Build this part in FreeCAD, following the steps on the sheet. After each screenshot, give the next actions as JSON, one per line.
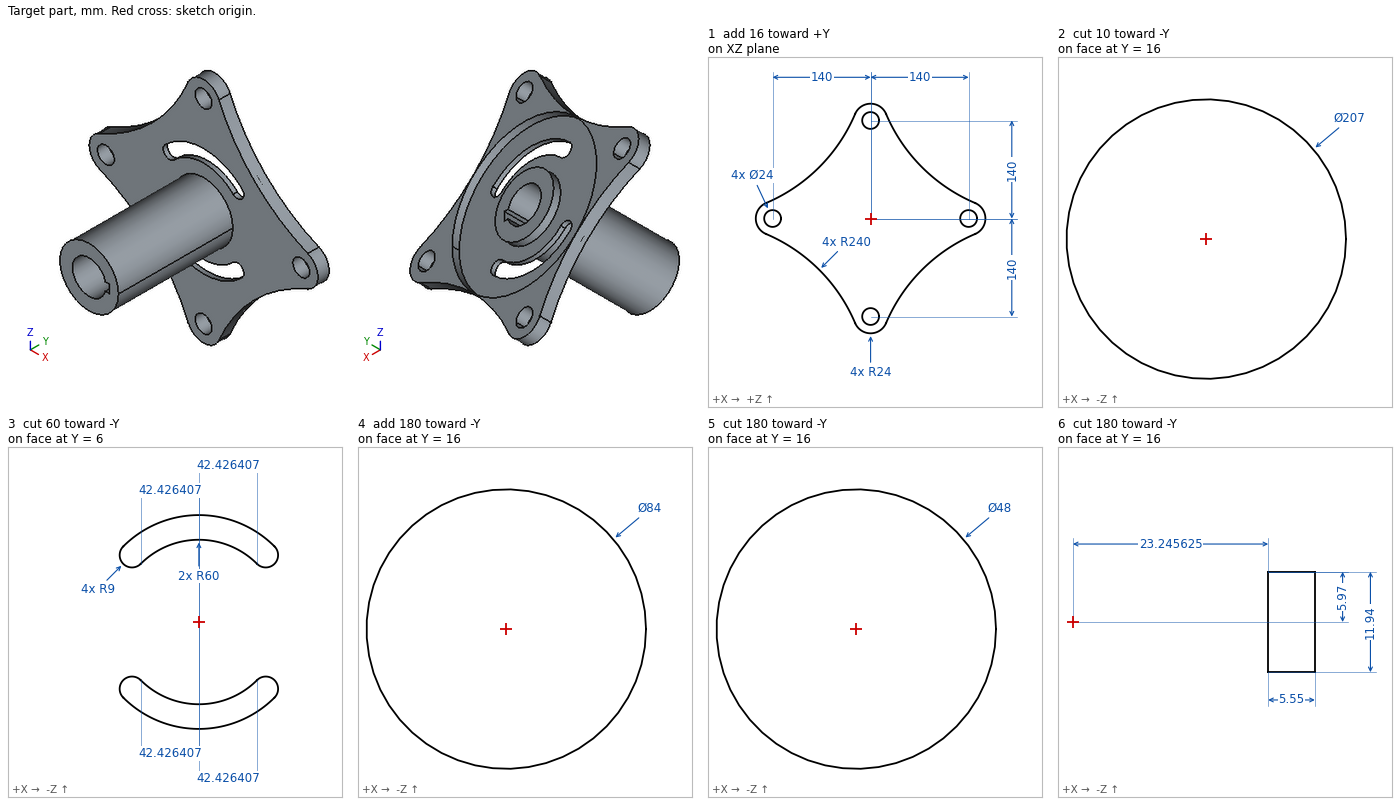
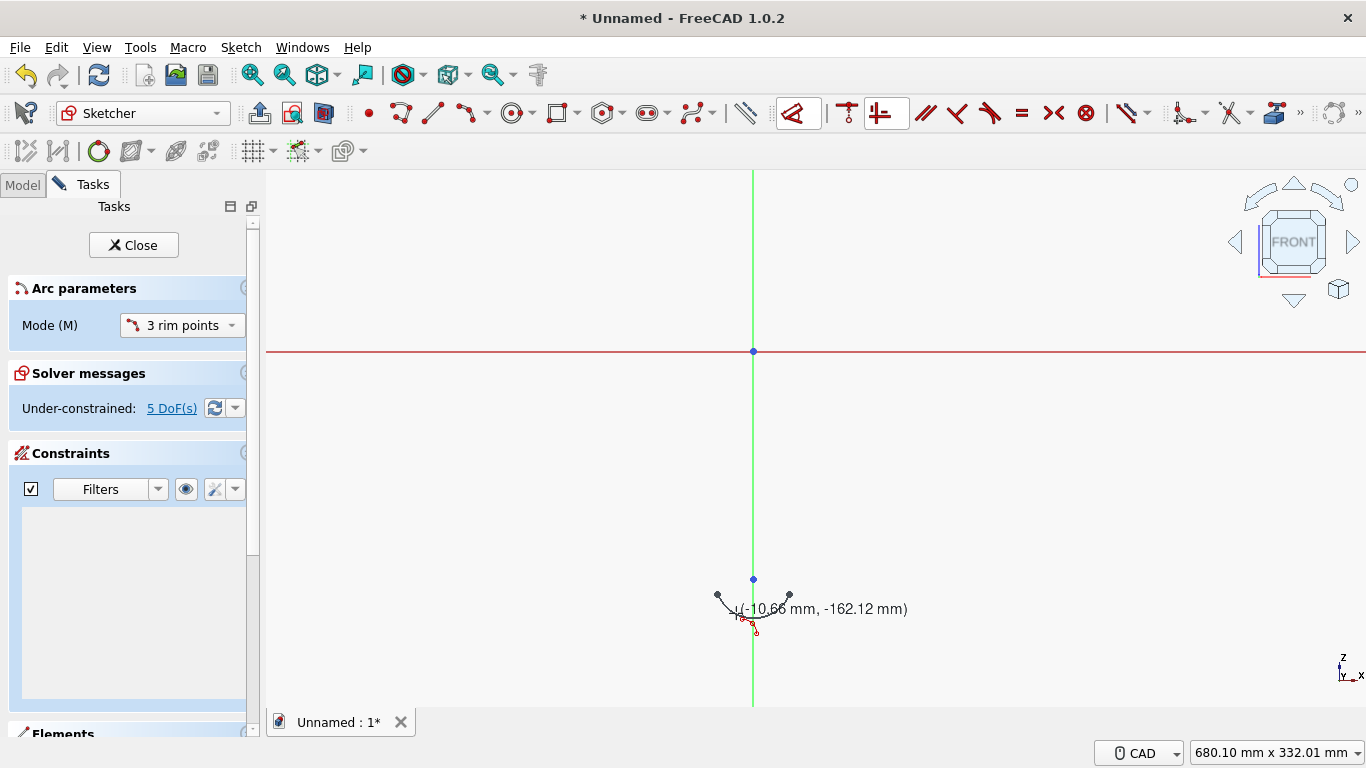
{"action": "left_click", "coordinate": [718, 594]}
{"action": "left_click", "coordinate": [512, 388]}
{"action": "left_click", "coordinate": [635, 470]}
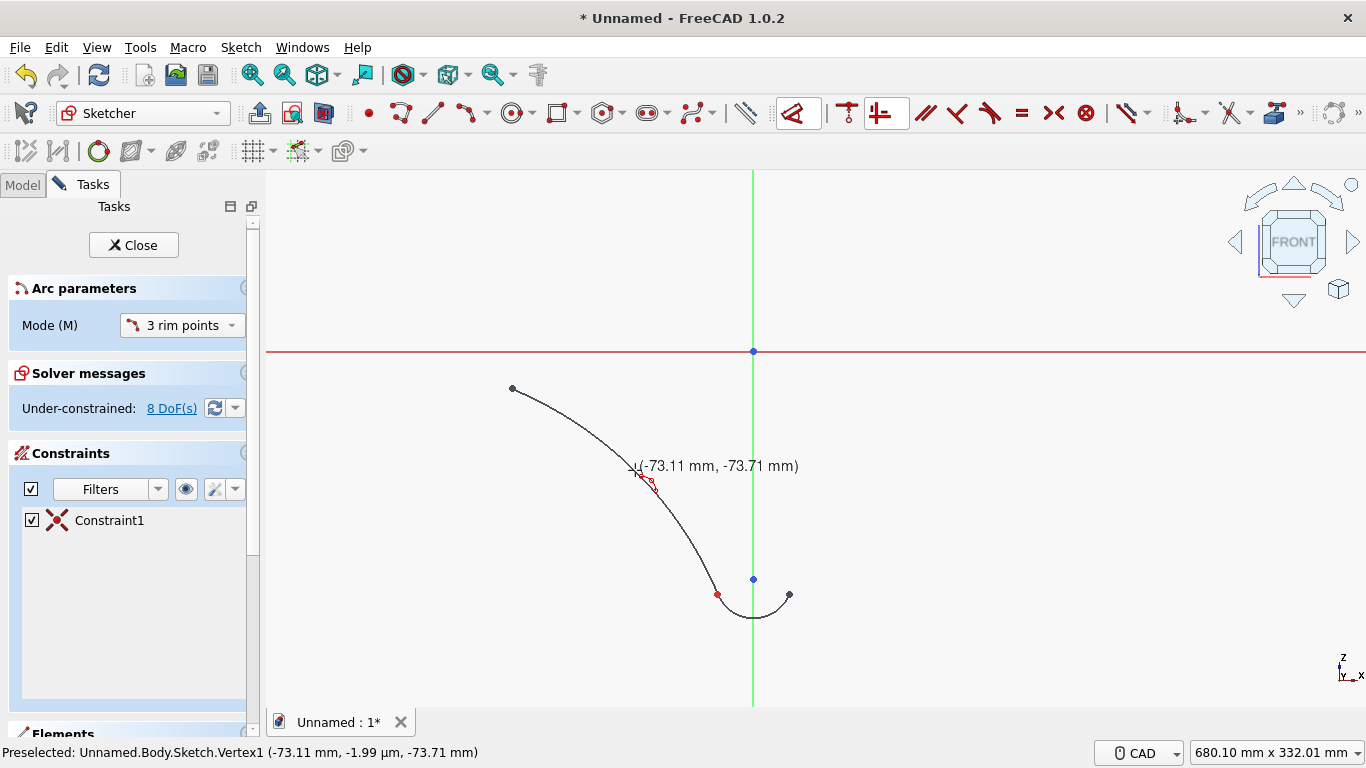
{"action": "left_click", "coordinate": [512, 389]}
{"action": "left_click", "coordinate": [512, 316]}
{"action": "left_click", "coordinate": [492, 334]}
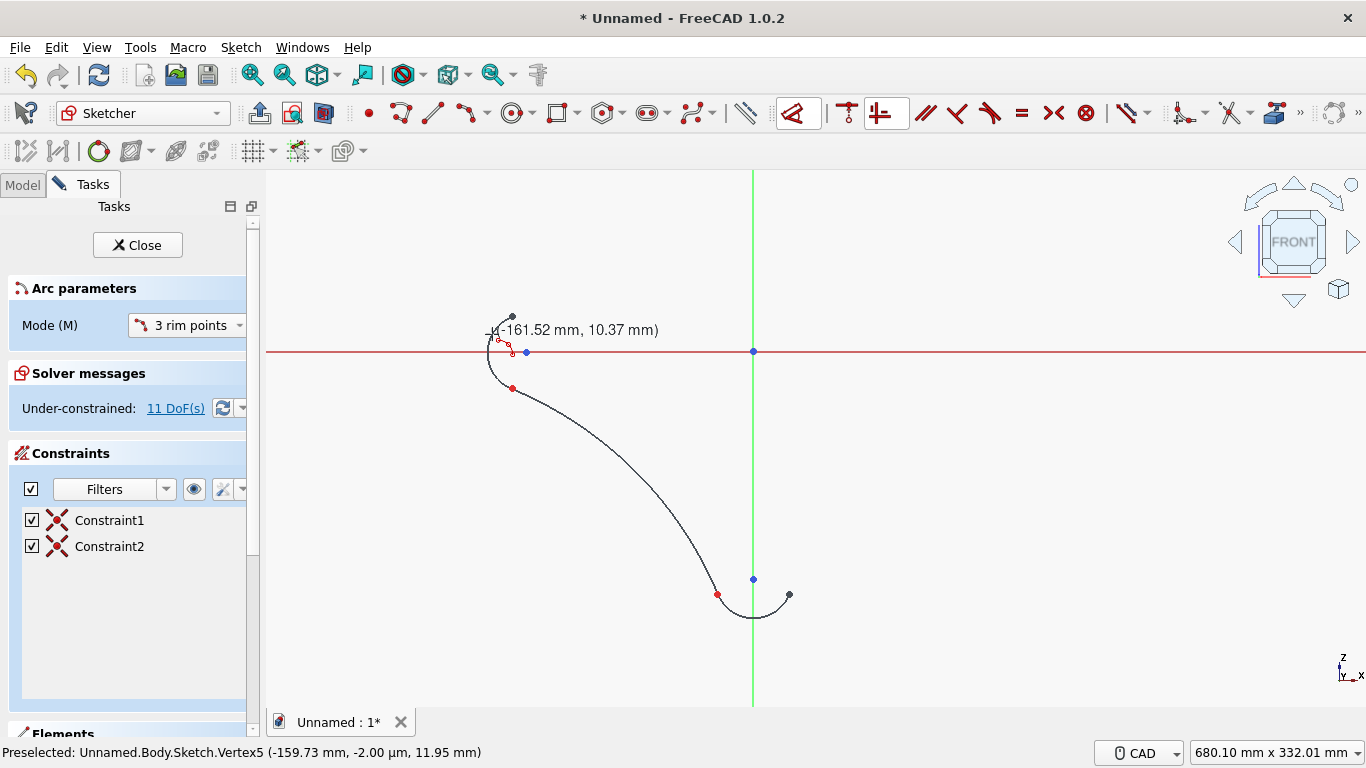
{"action": "left_click", "coordinate": [512, 317]}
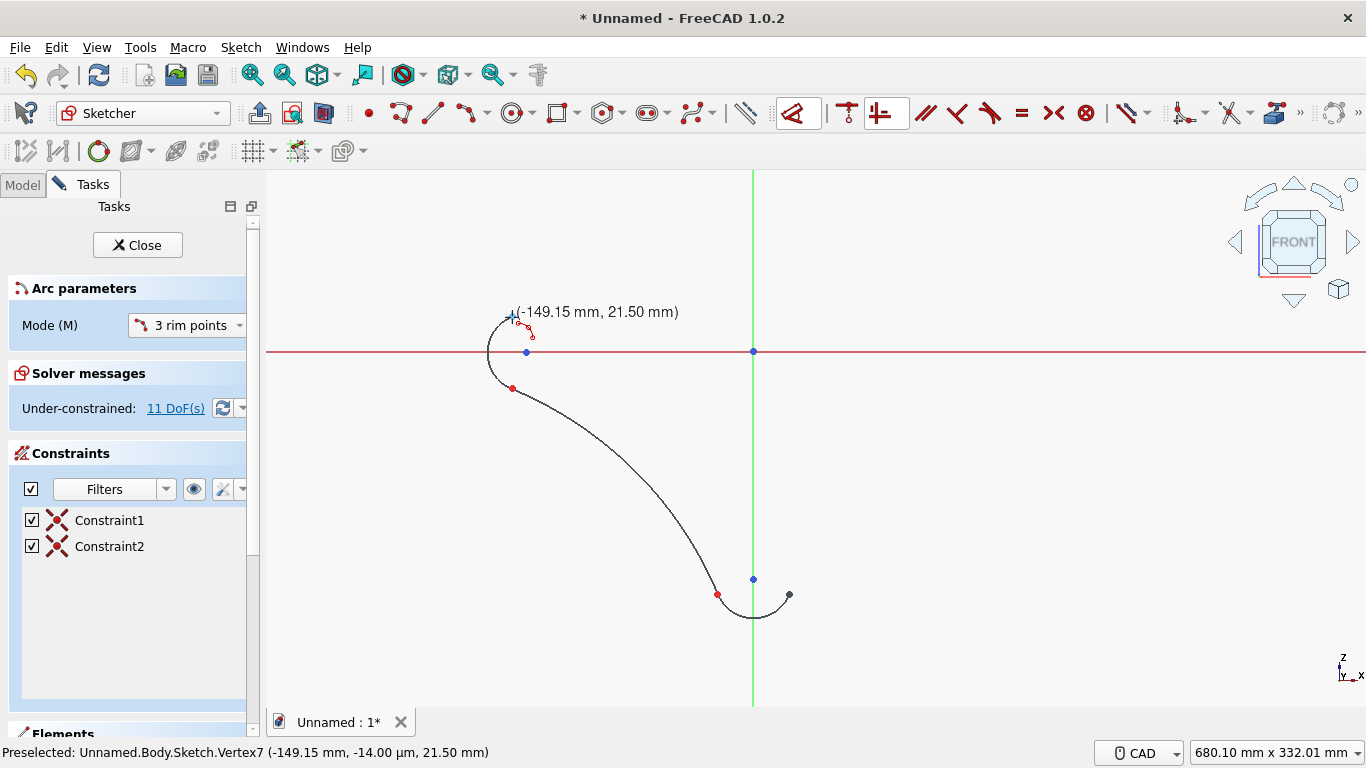
{"action": "scroll", "coordinate": [736, 615], "scroll_direction": "down", "scroll_amount": 2}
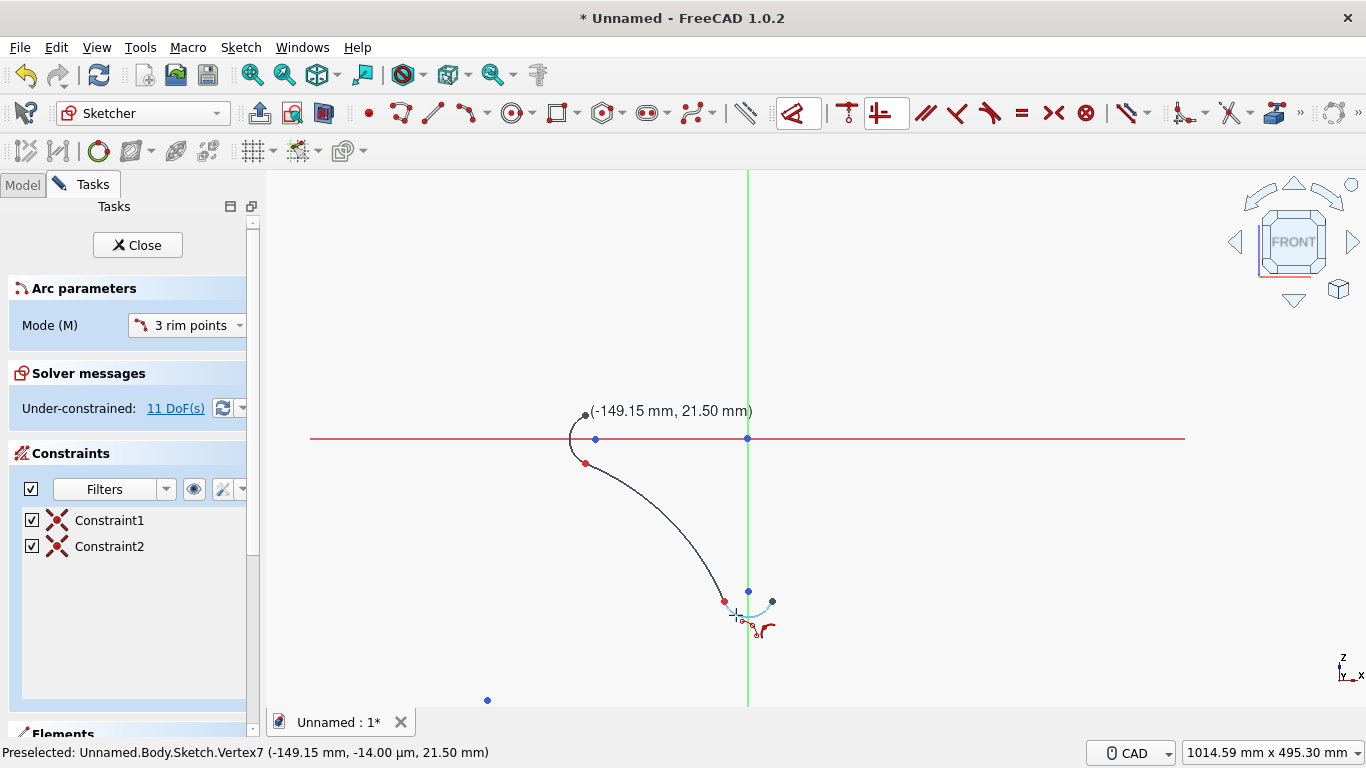
{"action": "left_click", "coordinate": [724, 277]}
{"action": "left_click", "coordinate": [668, 359]}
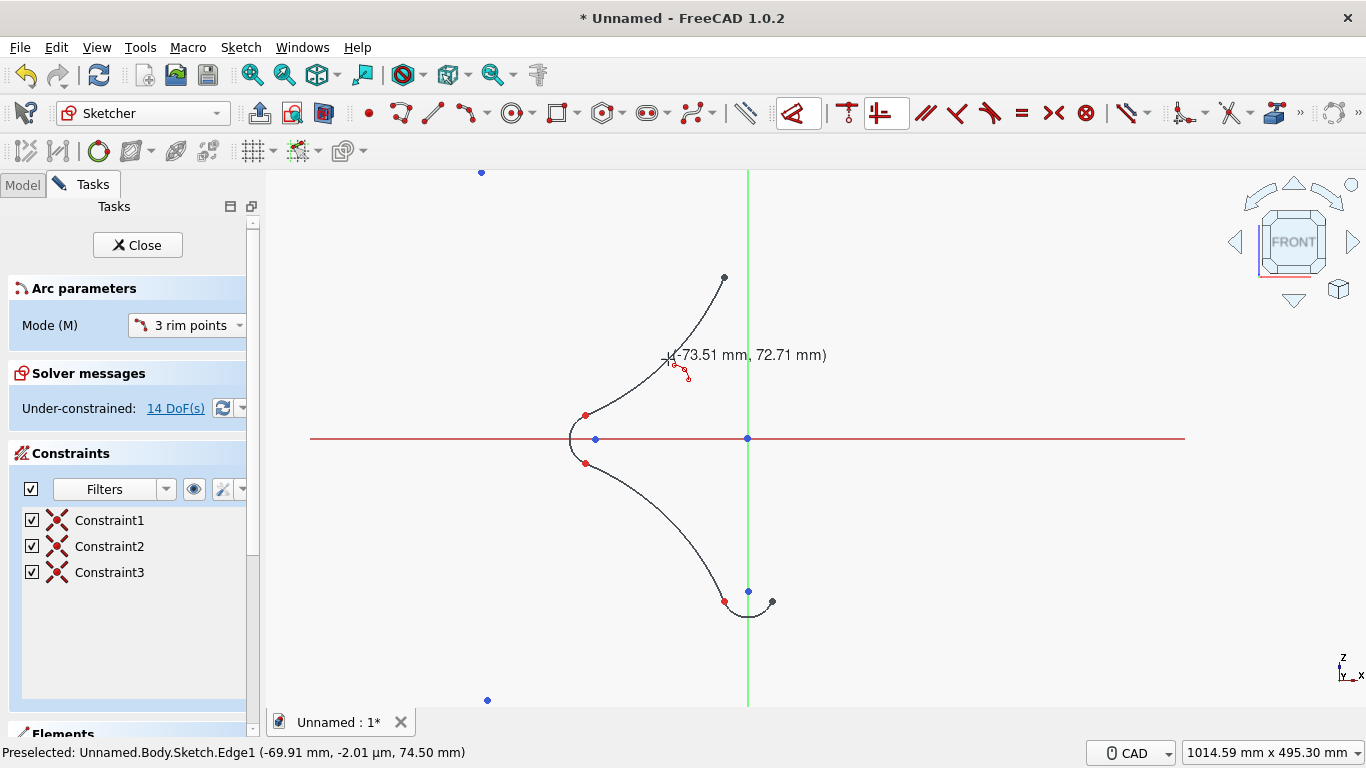
{"action": "left_click", "coordinate": [724, 278]}
{"action": "left_click", "coordinate": [772, 277]}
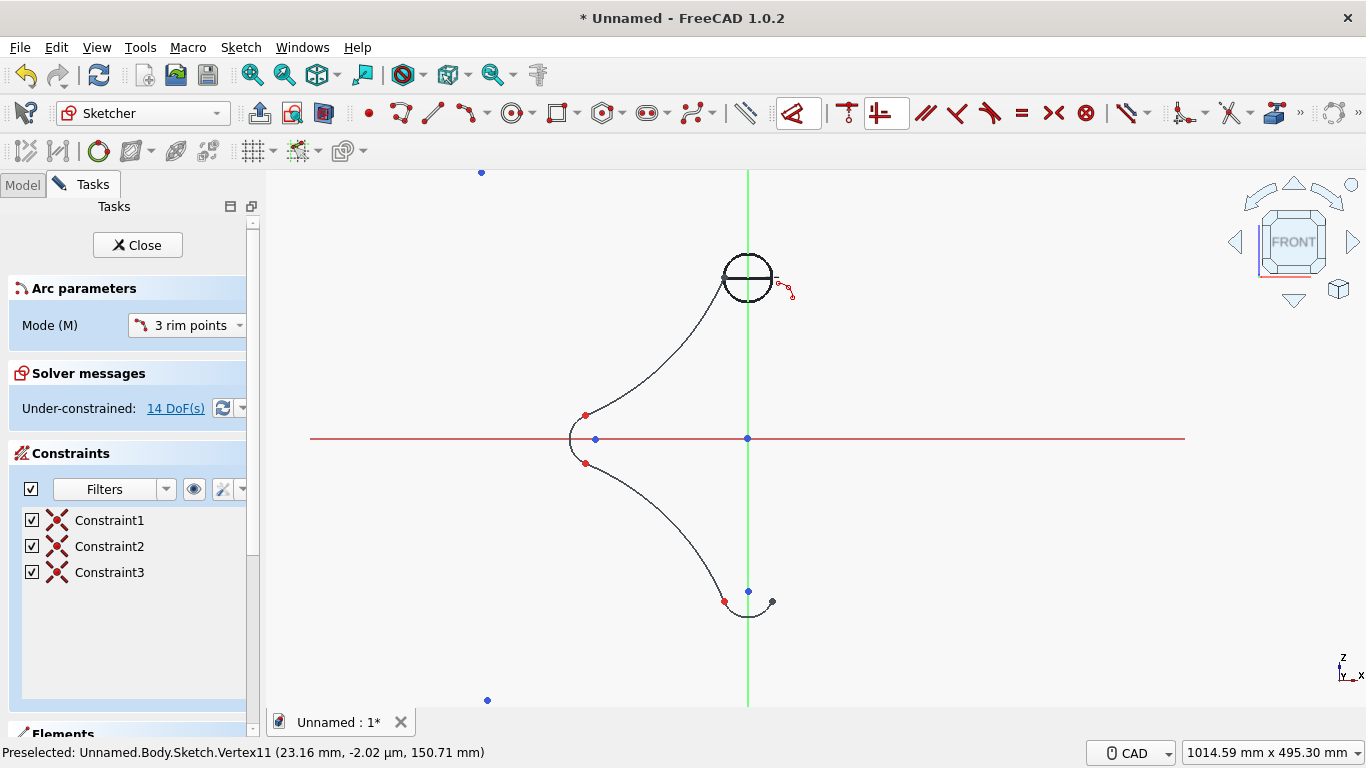
{"action": "scroll", "coordinate": [759, 264], "scroll_direction": "up", "scroll_amount": 2}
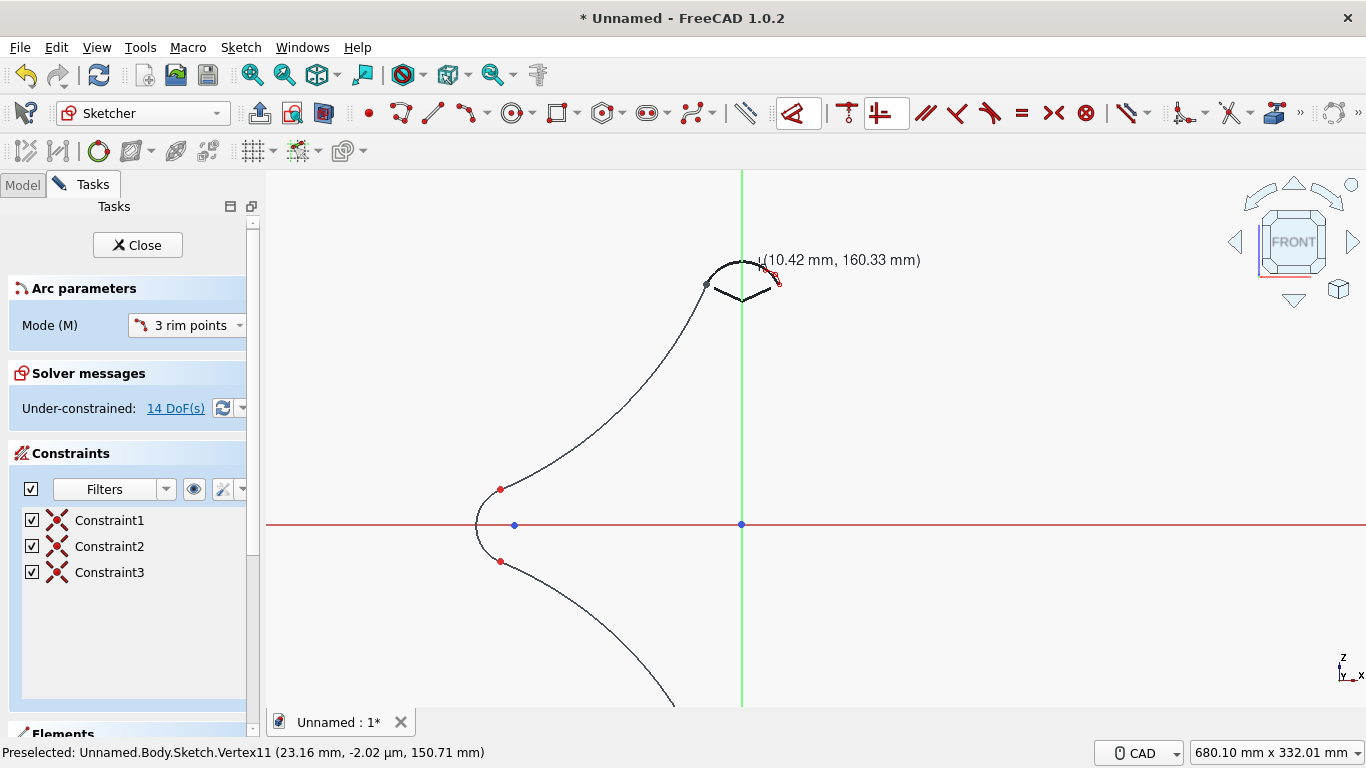
{"action": "left_click", "coordinate": [759, 264]}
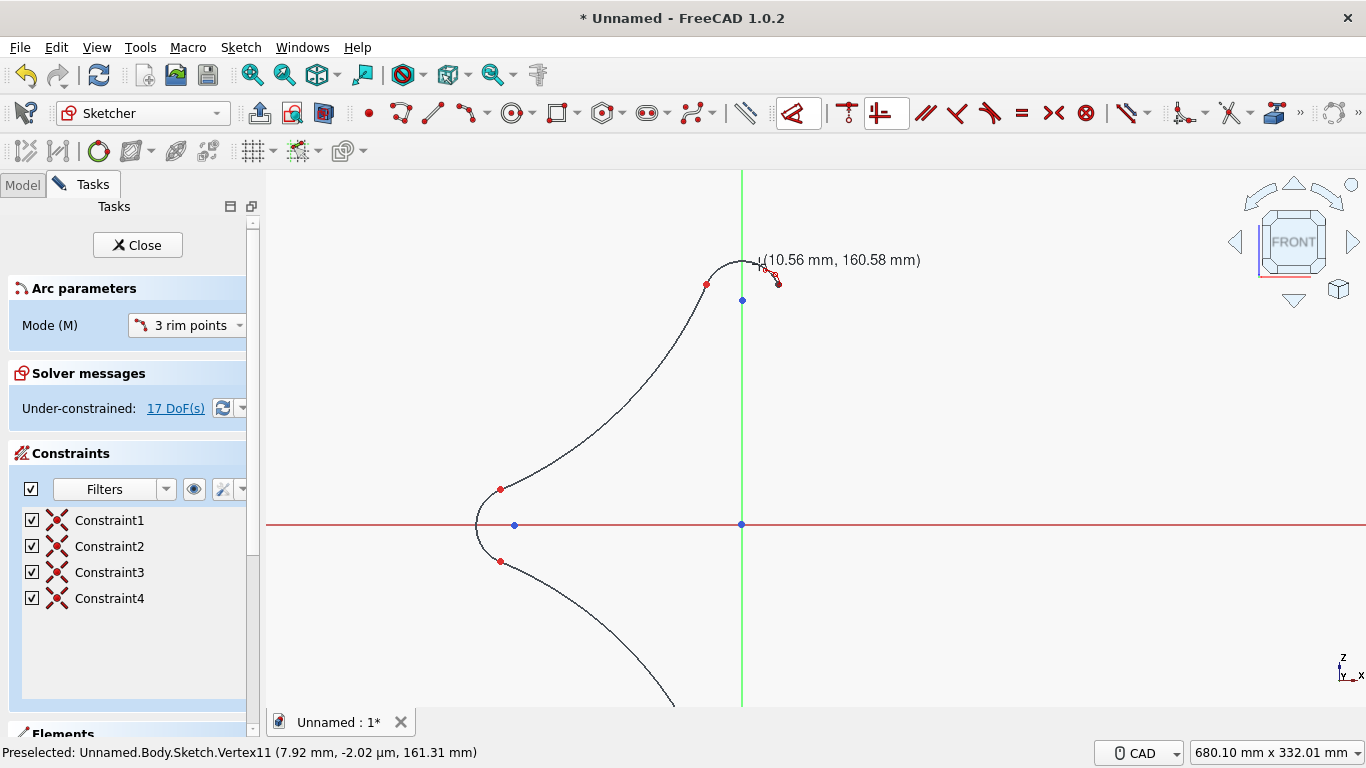
{"action": "left_click", "coordinate": [778, 285]}
{"action": "left_click", "coordinate": [984, 489]}
{"action": "left_click", "coordinate": [861, 406]}